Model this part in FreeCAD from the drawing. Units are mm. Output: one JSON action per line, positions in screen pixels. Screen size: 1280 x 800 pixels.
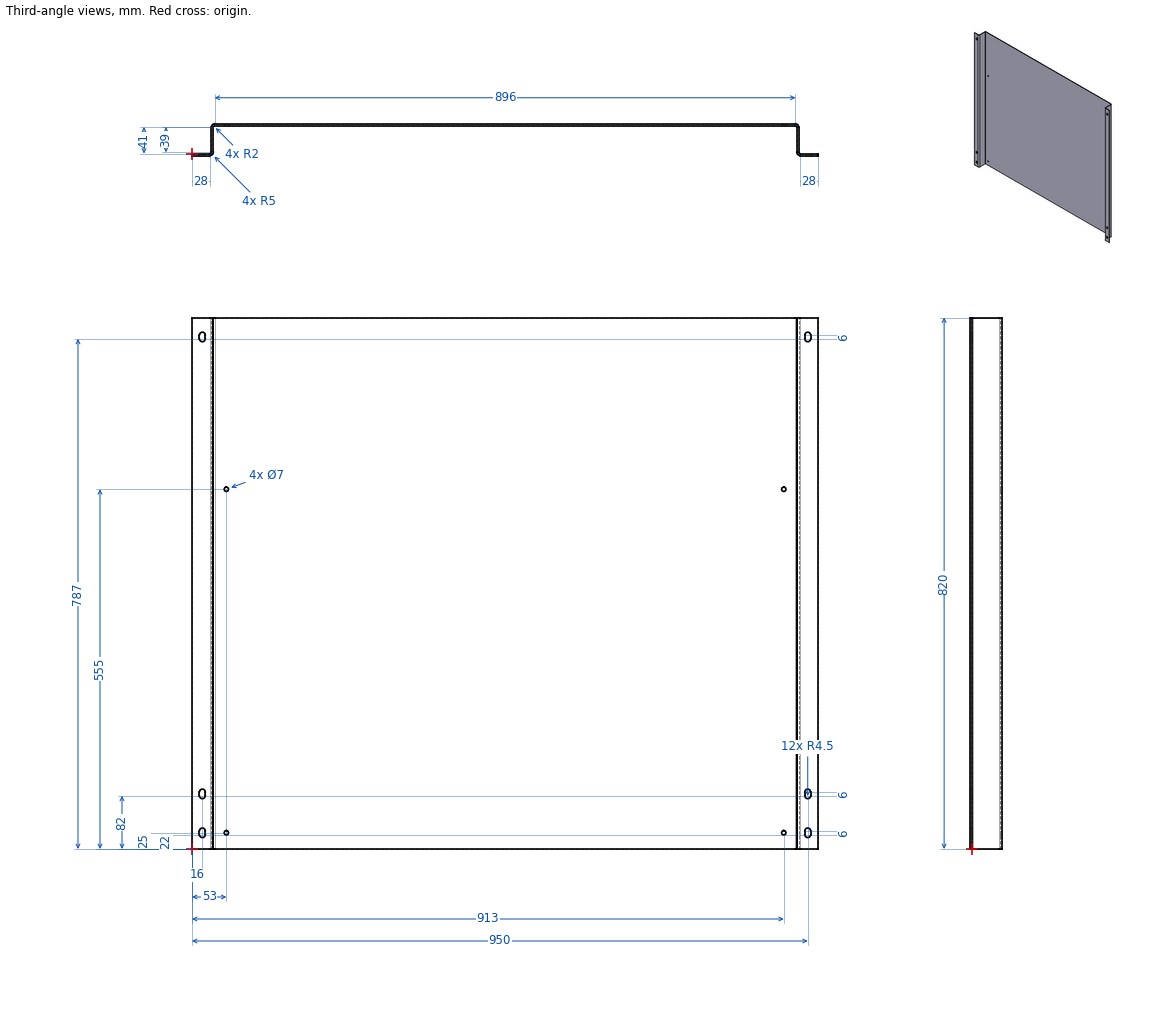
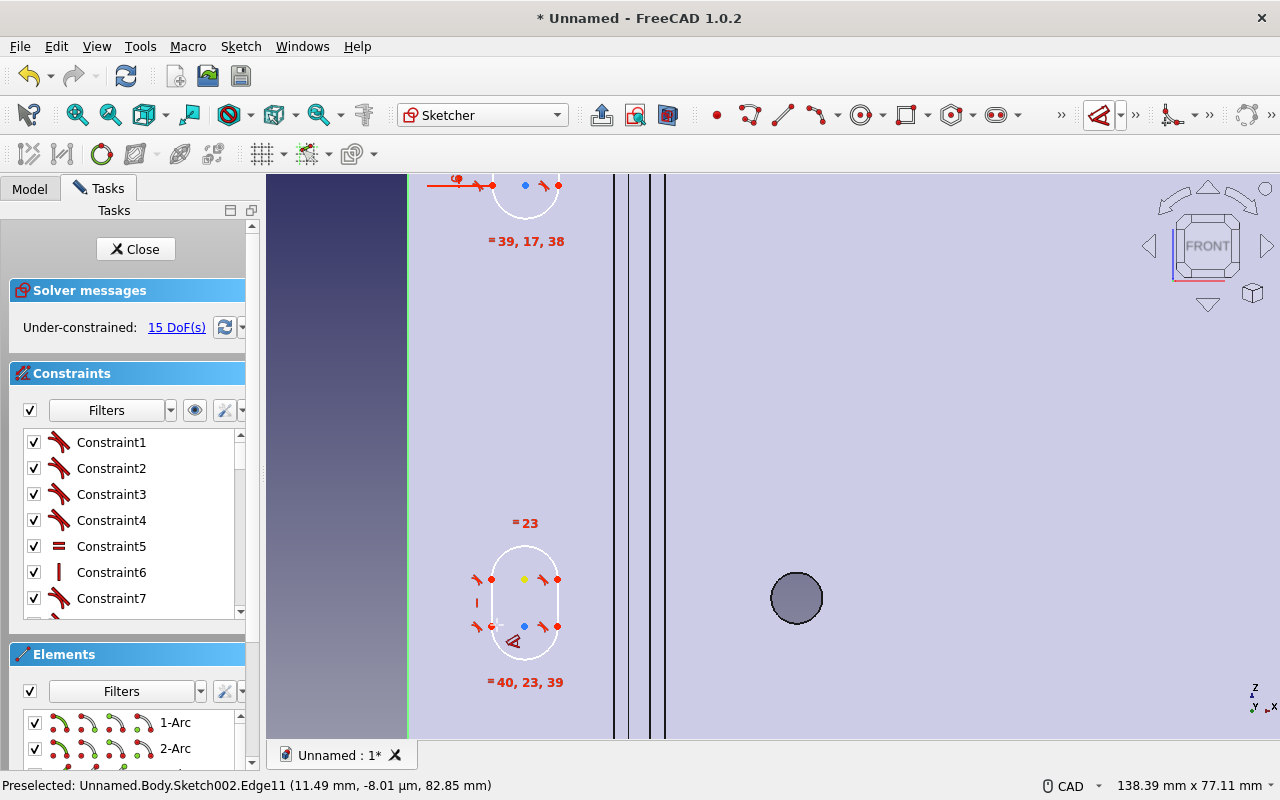
{"action": "left_click", "coordinate": [492, 612]}
{"action": "left_click", "coordinate": [458, 603]}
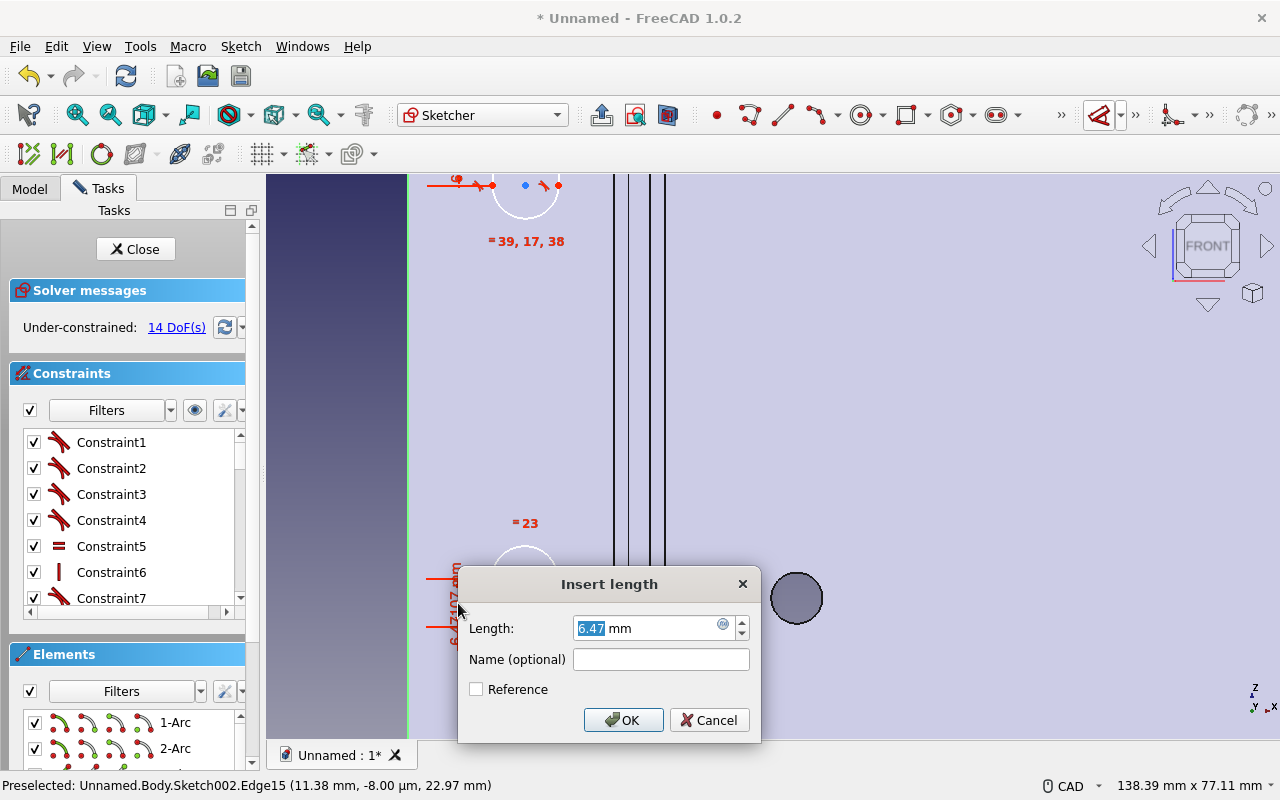
{"action": "type", "text": "6"}
{"action": "key", "text": "Return"}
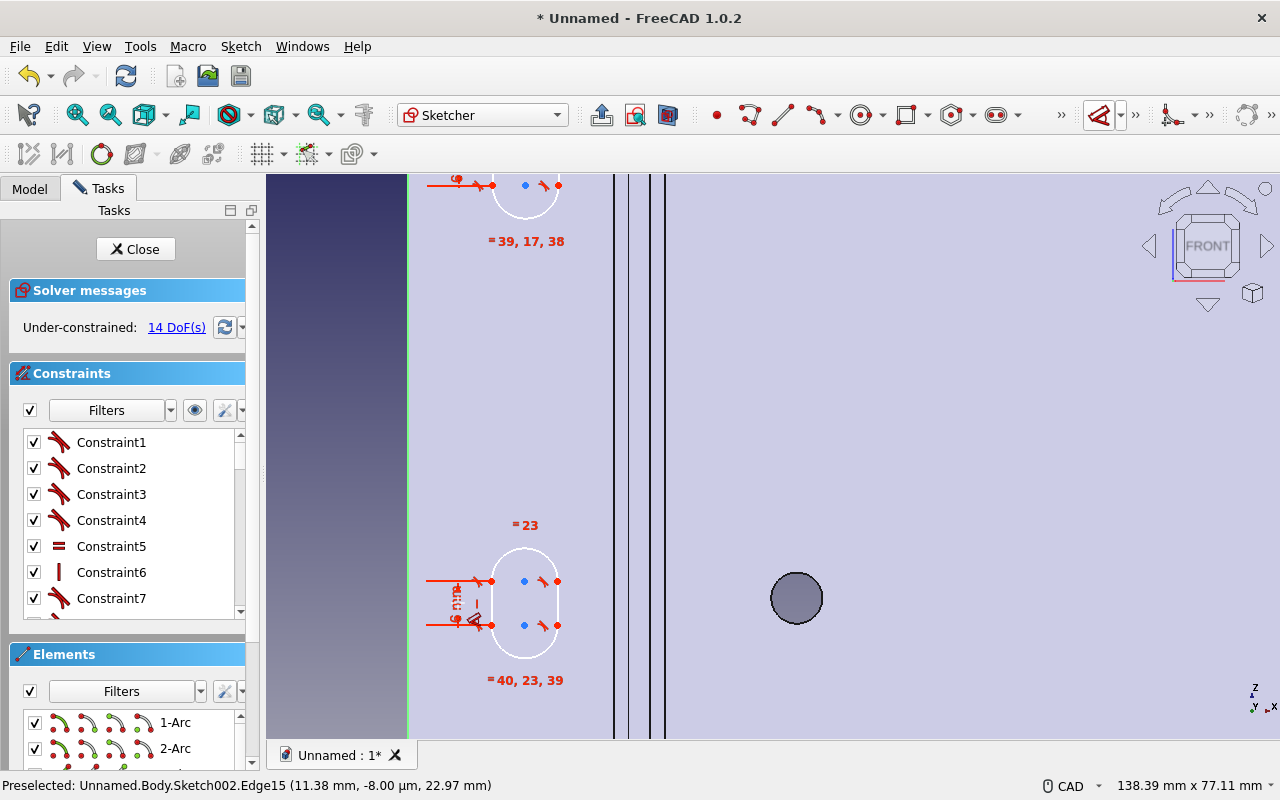
{"action": "scroll", "coordinate": [497, 625], "scroll_direction": "down", "scroll_amount": 14}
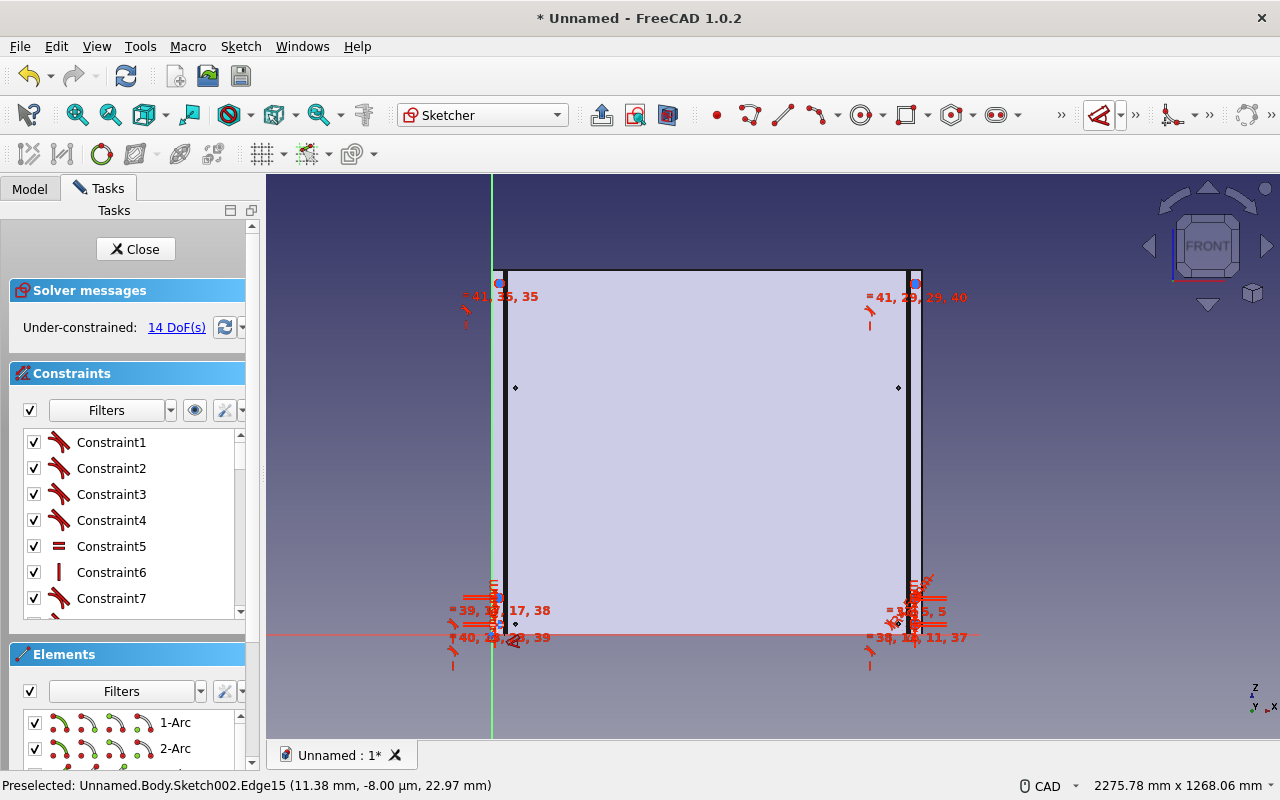
{"action": "scroll", "coordinate": [913, 284], "scroll_direction": "up", "scroll_amount": 14}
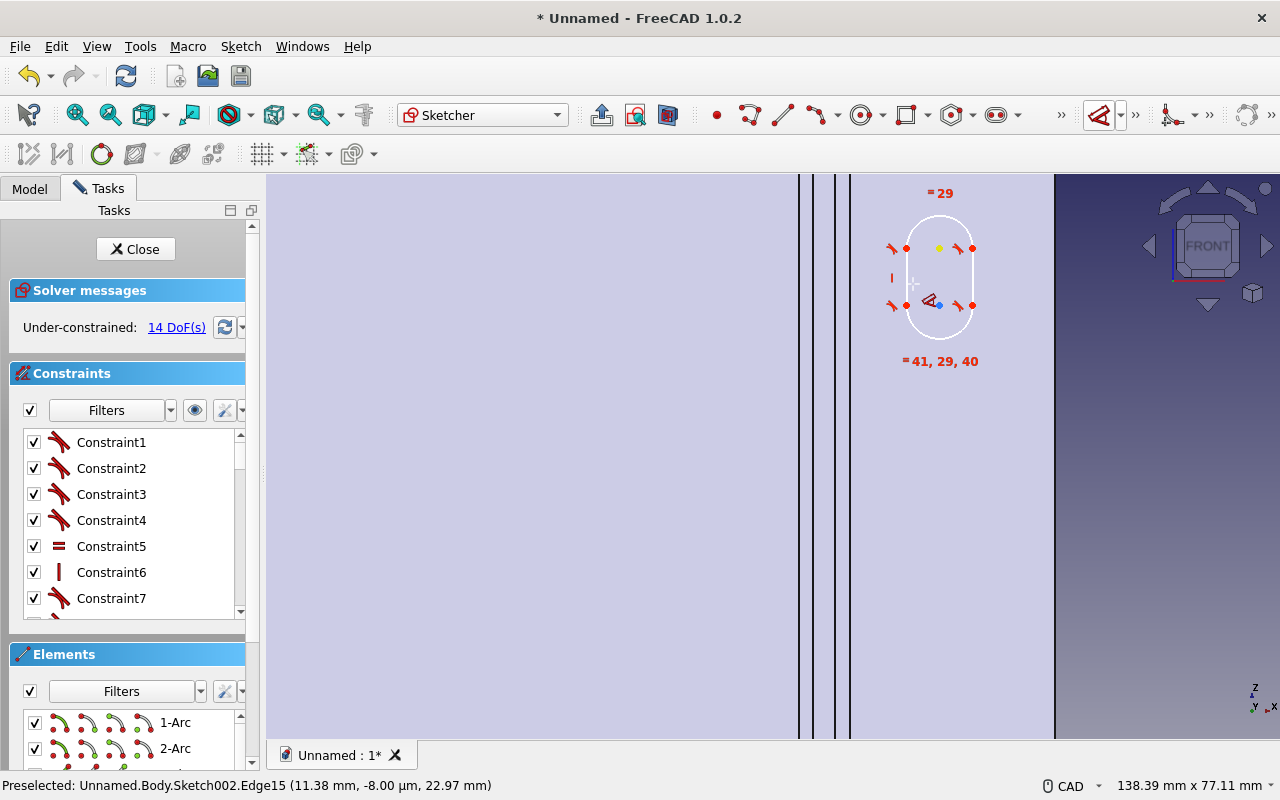
{"action": "left_click", "coordinate": [907, 289]}
{"action": "left_click", "coordinate": [941, 277]}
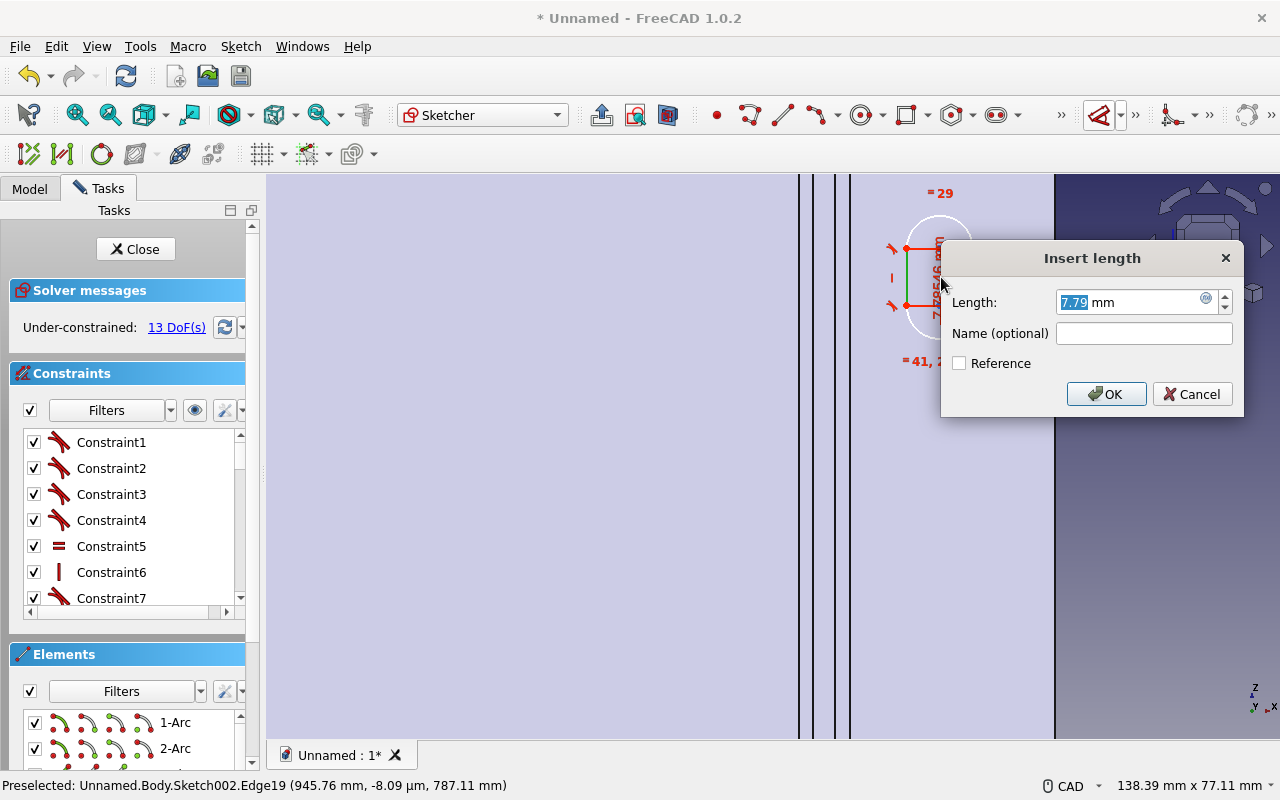
{"action": "type", "text": "6"}
{"action": "key", "text": "Return"}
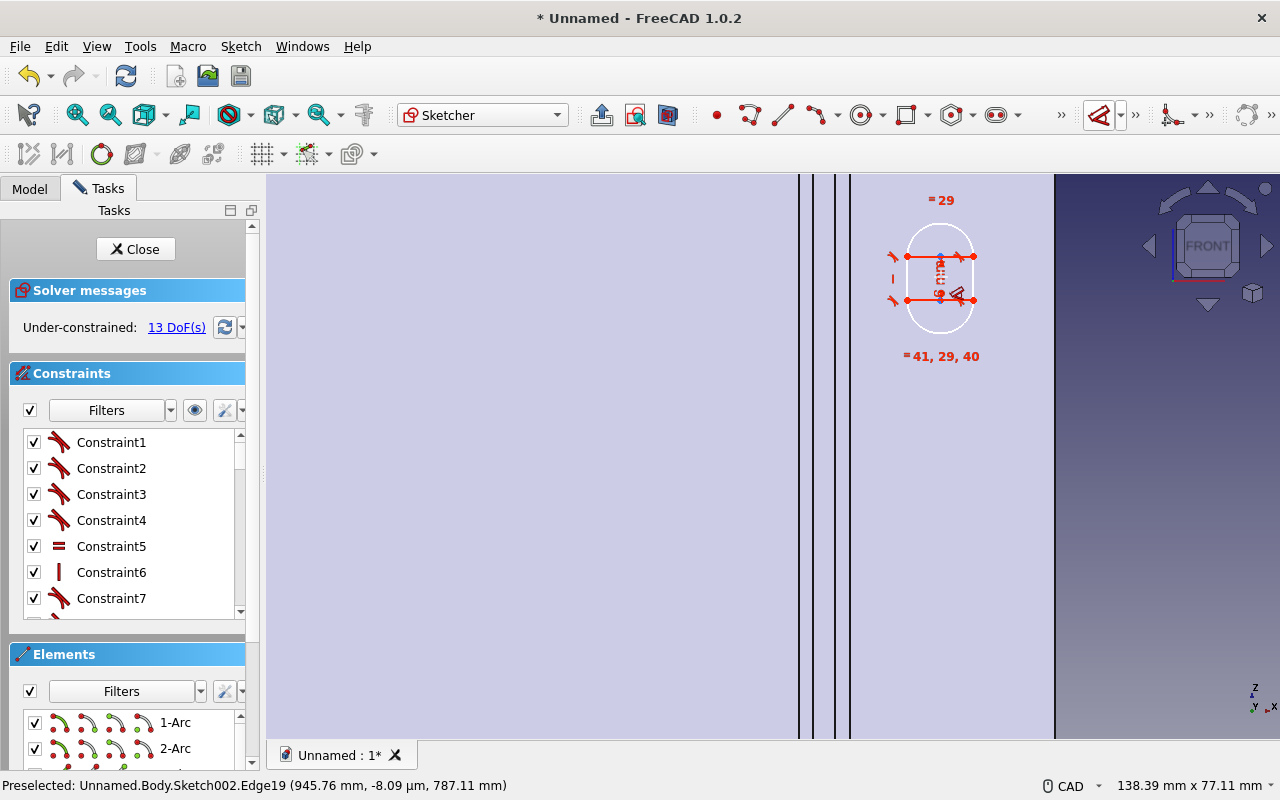
{"action": "scroll", "coordinate": [914, 283], "scroll_direction": "down", "scroll_amount": 14}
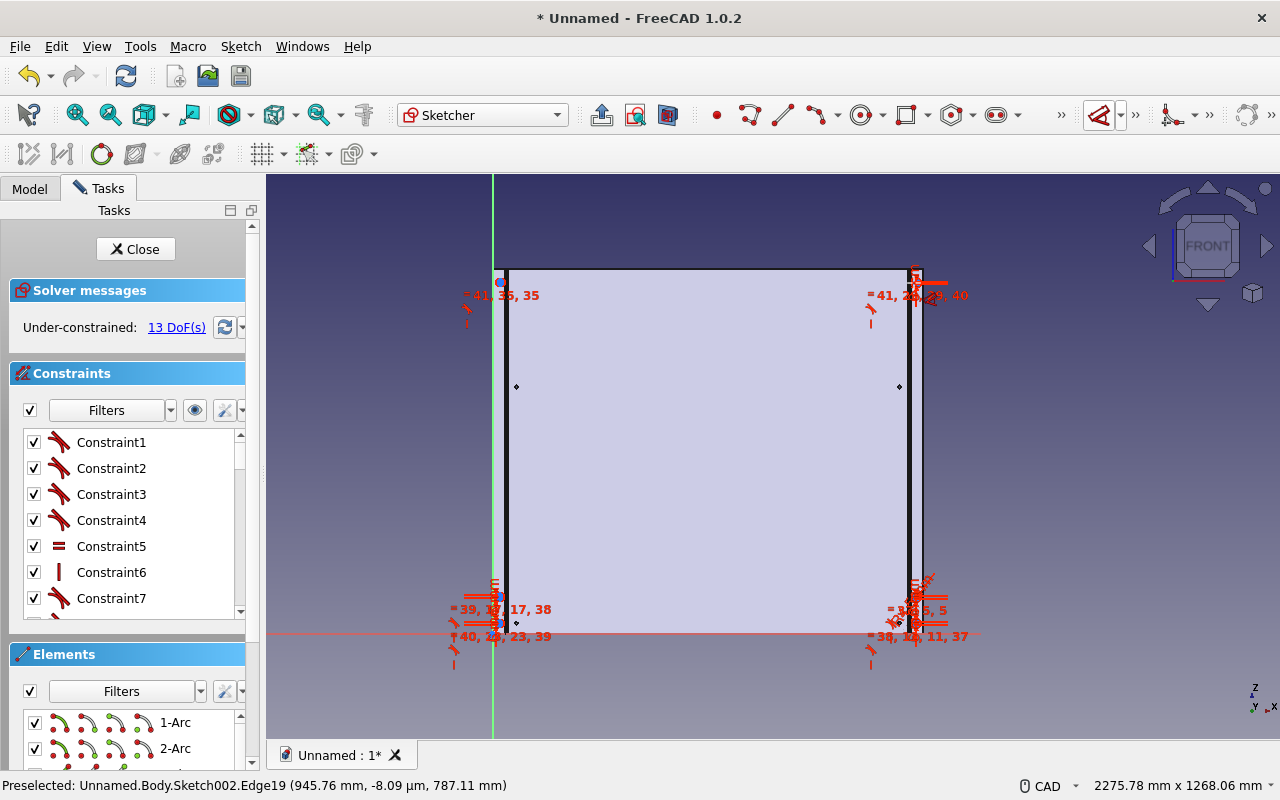
{"action": "scroll", "coordinate": [498, 283], "scroll_direction": "up", "scroll_amount": 14}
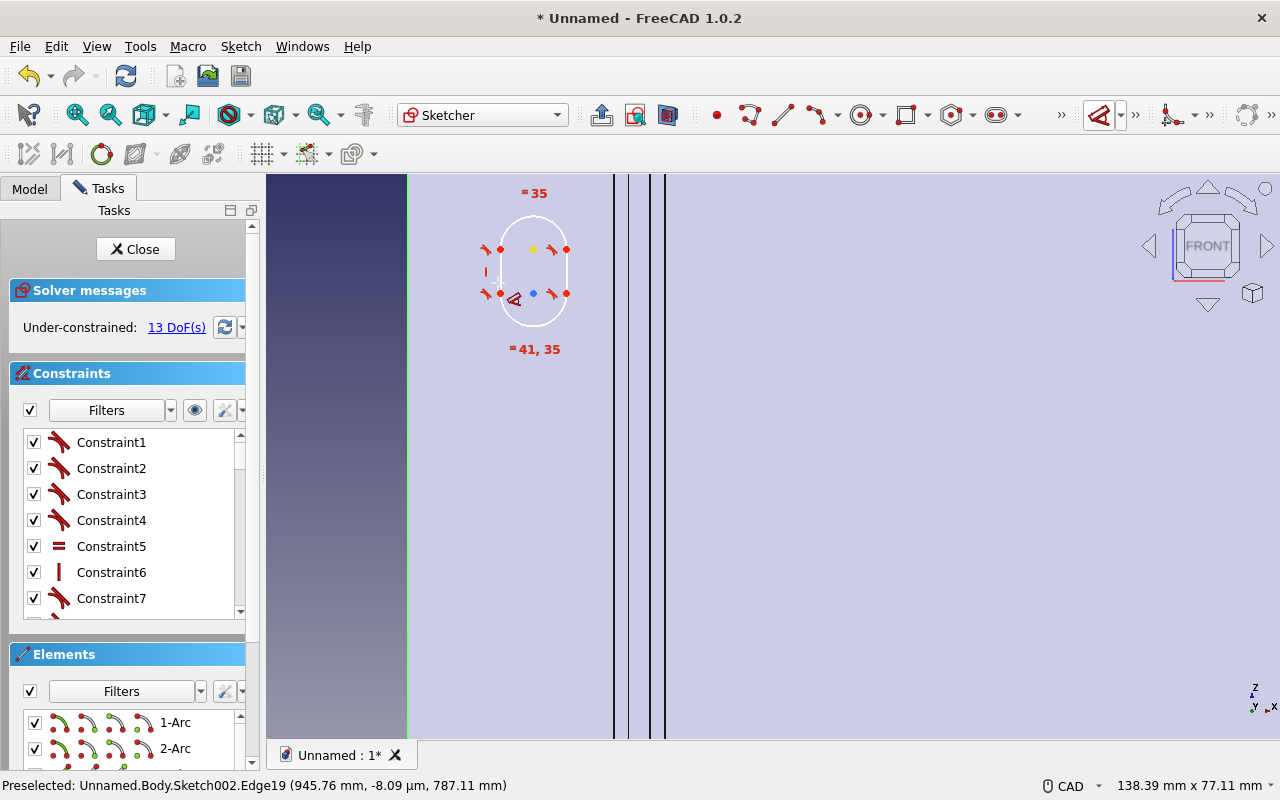
{"action": "left_click", "coordinate": [501, 280]}
{"action": "left_click", "coordinate": [467, 271]}